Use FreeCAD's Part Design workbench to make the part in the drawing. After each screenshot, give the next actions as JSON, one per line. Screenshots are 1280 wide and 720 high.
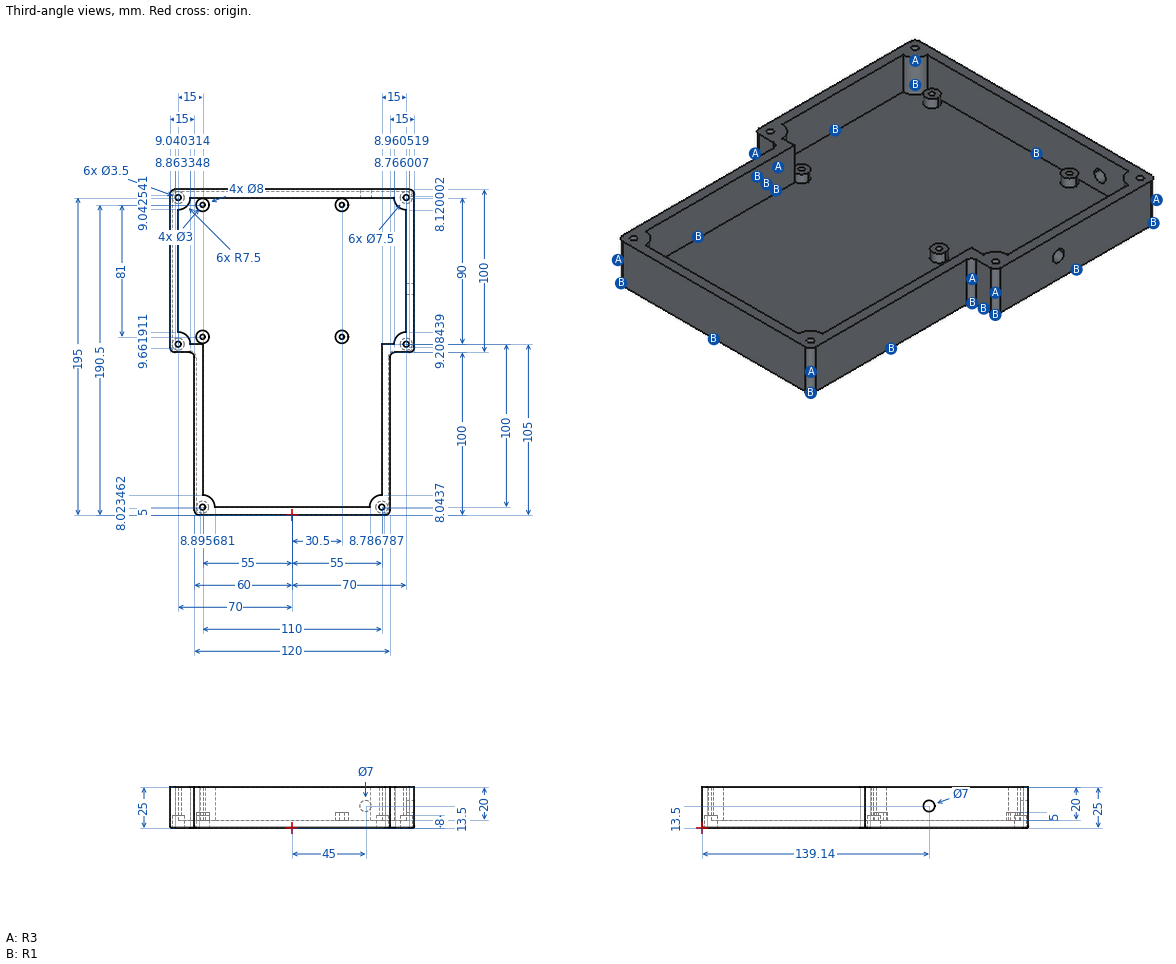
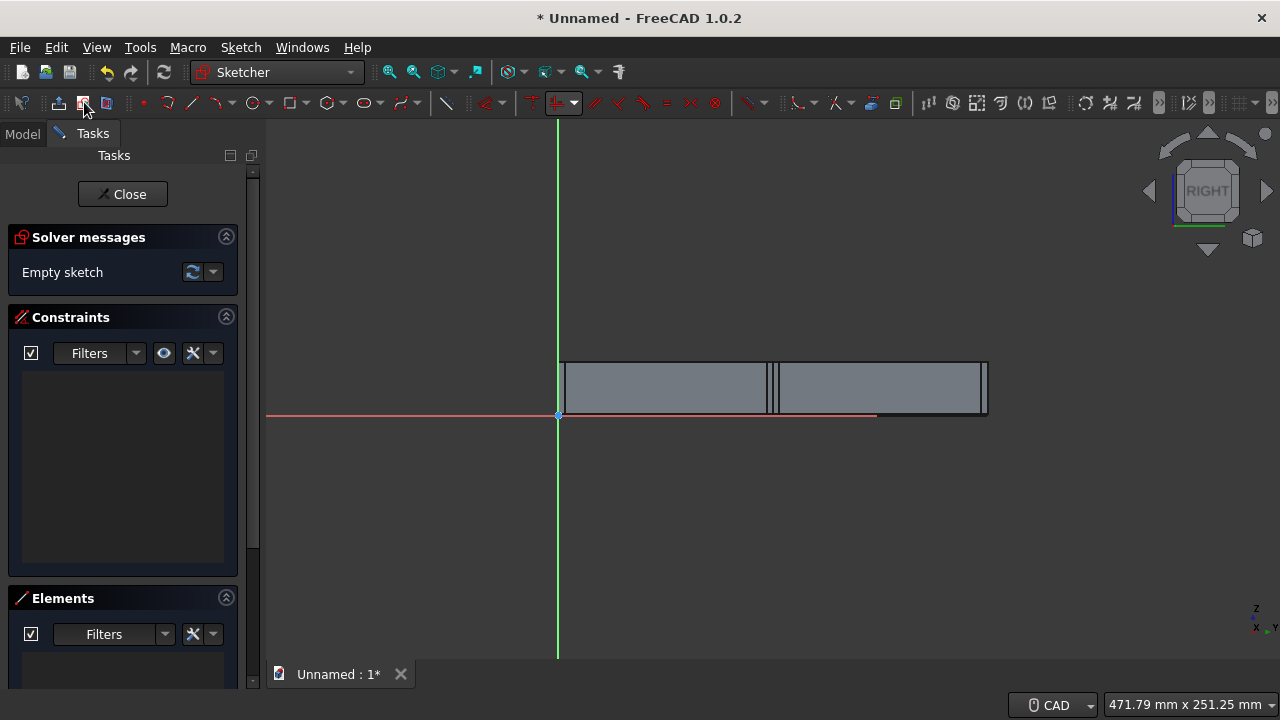
{"action": "scroll", "coordinate": [865, 387], "scroll_direction": "up", "scroll_amount": 15}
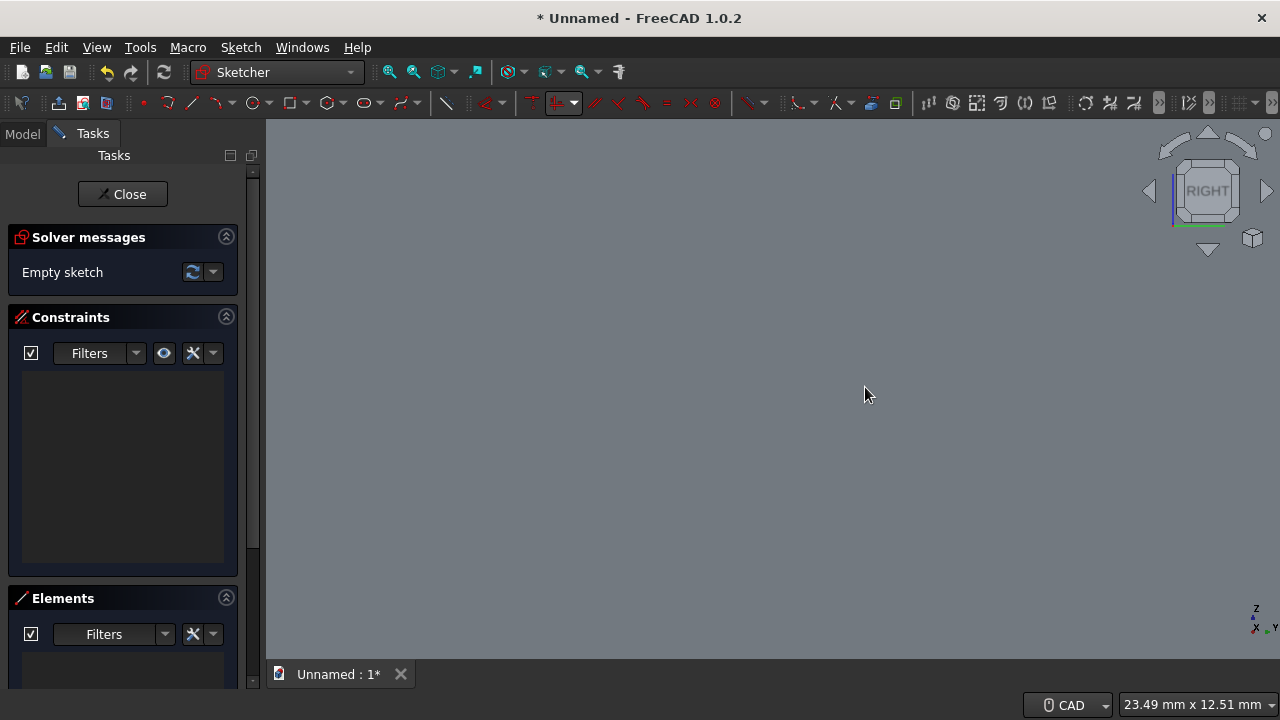
{"action": "left_click", "coordinate": [254, 104]}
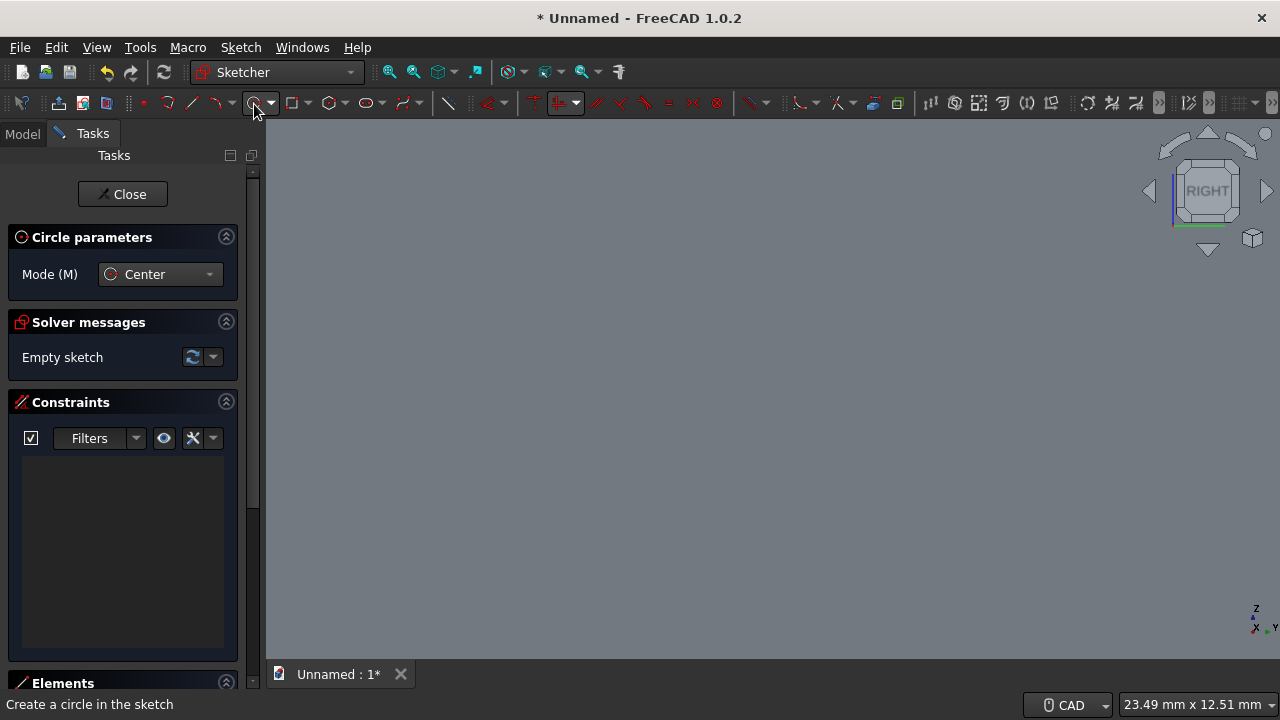
{"action": "left_click", "coordinate": [695, 375]}
{"action": "mouse_move", "coordinate": [802, 268]}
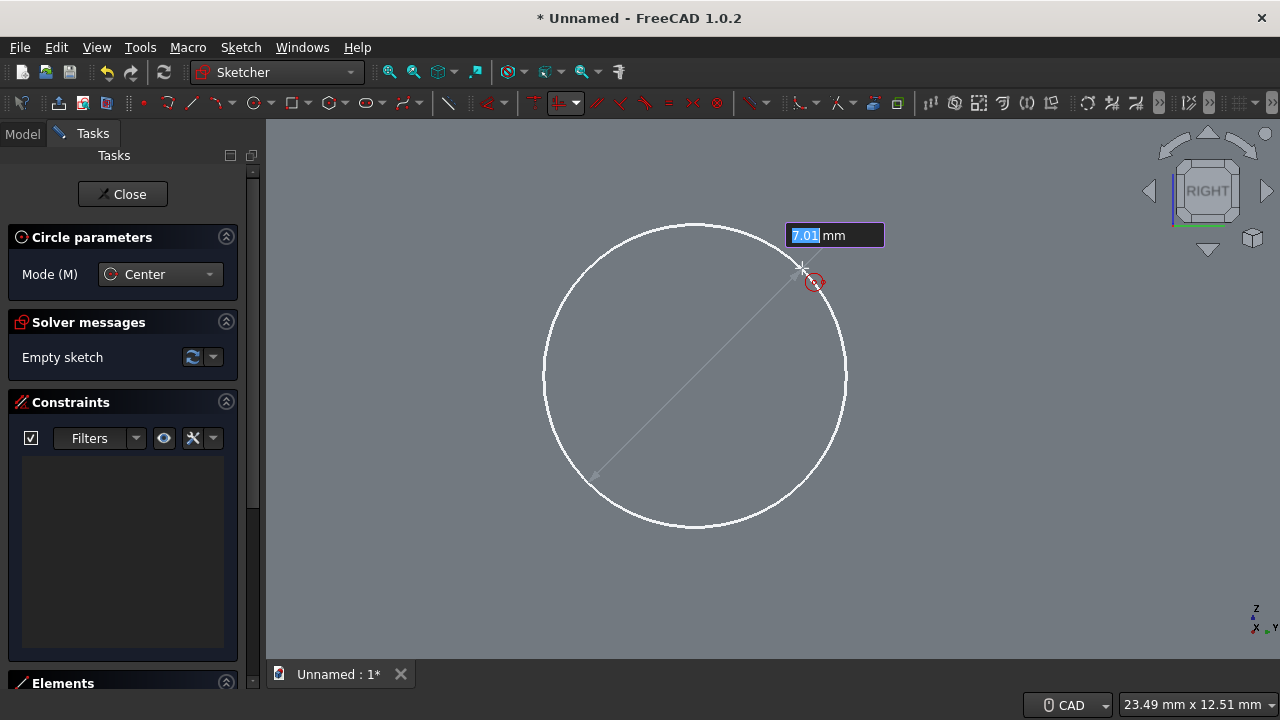
{"action": "type", "text": "7"}
{"action": "key", "text": "Return"}
{"action": "key", "text": "Escape"}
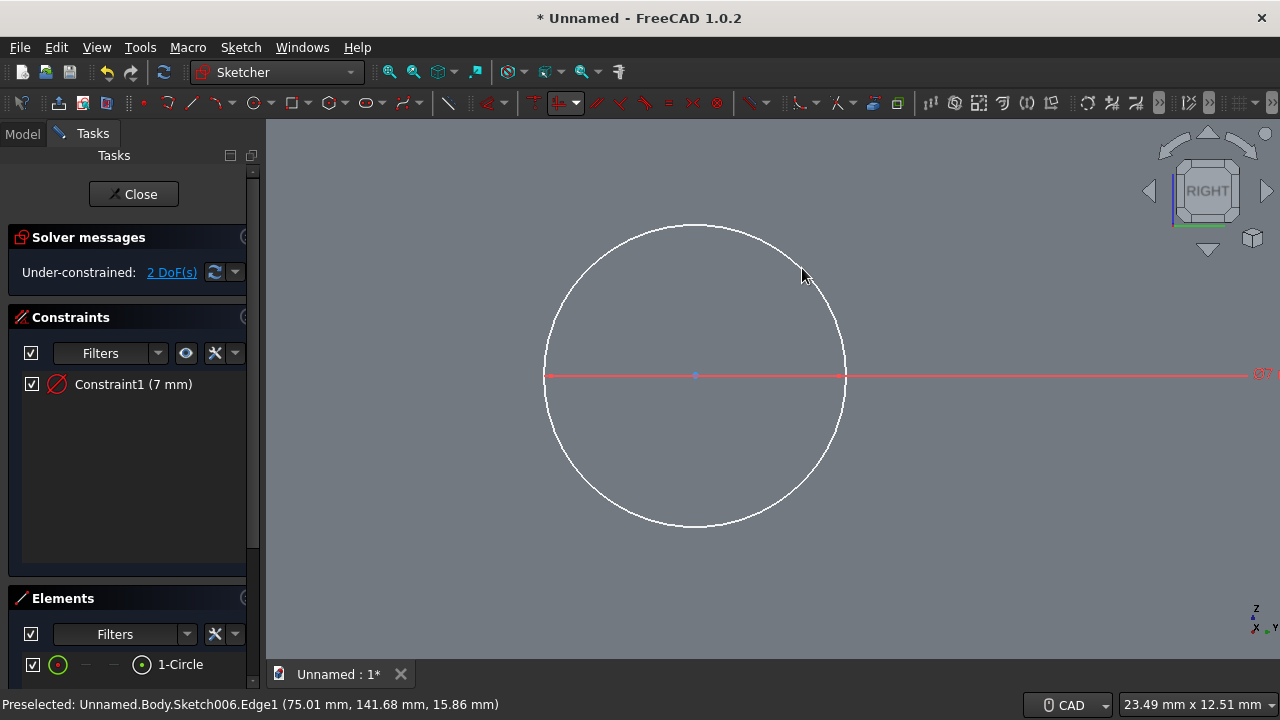
{"action": "left_click", "coordinate": [488, 104]}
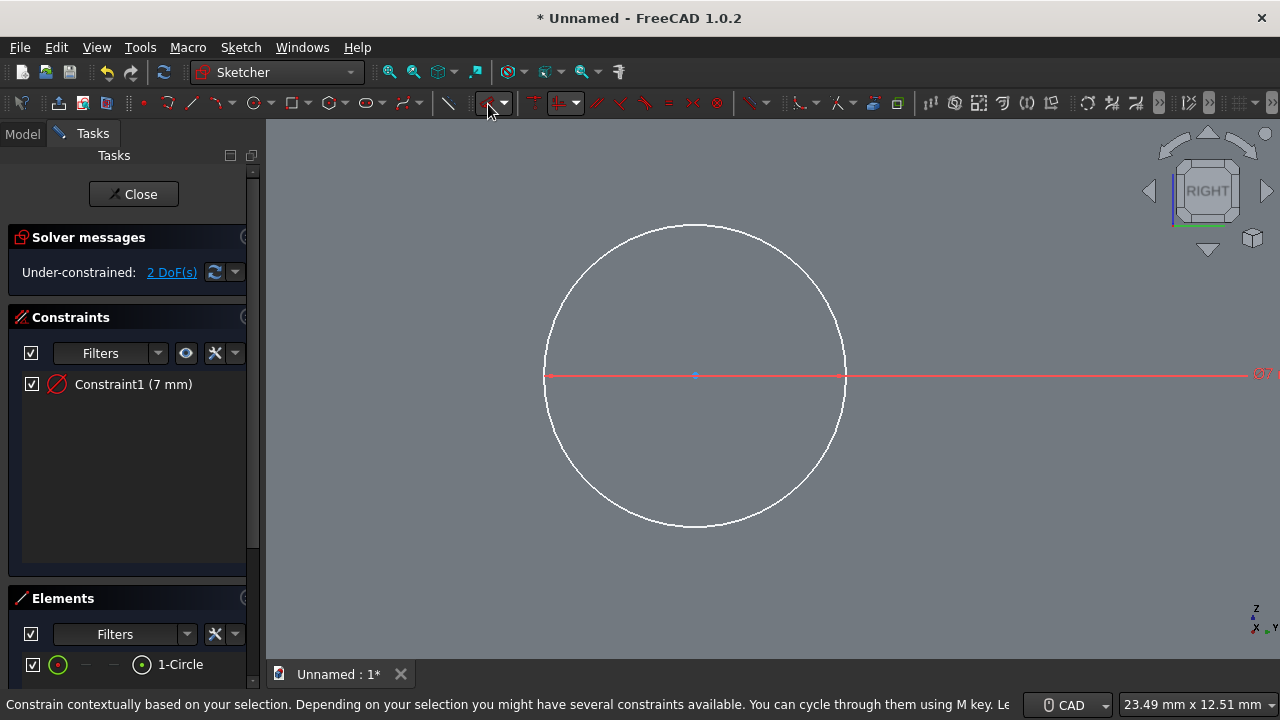
{"action": "left_click", "coordinate": [695, 376]}
{"action": "left_click", "coordinate": [729, 504]}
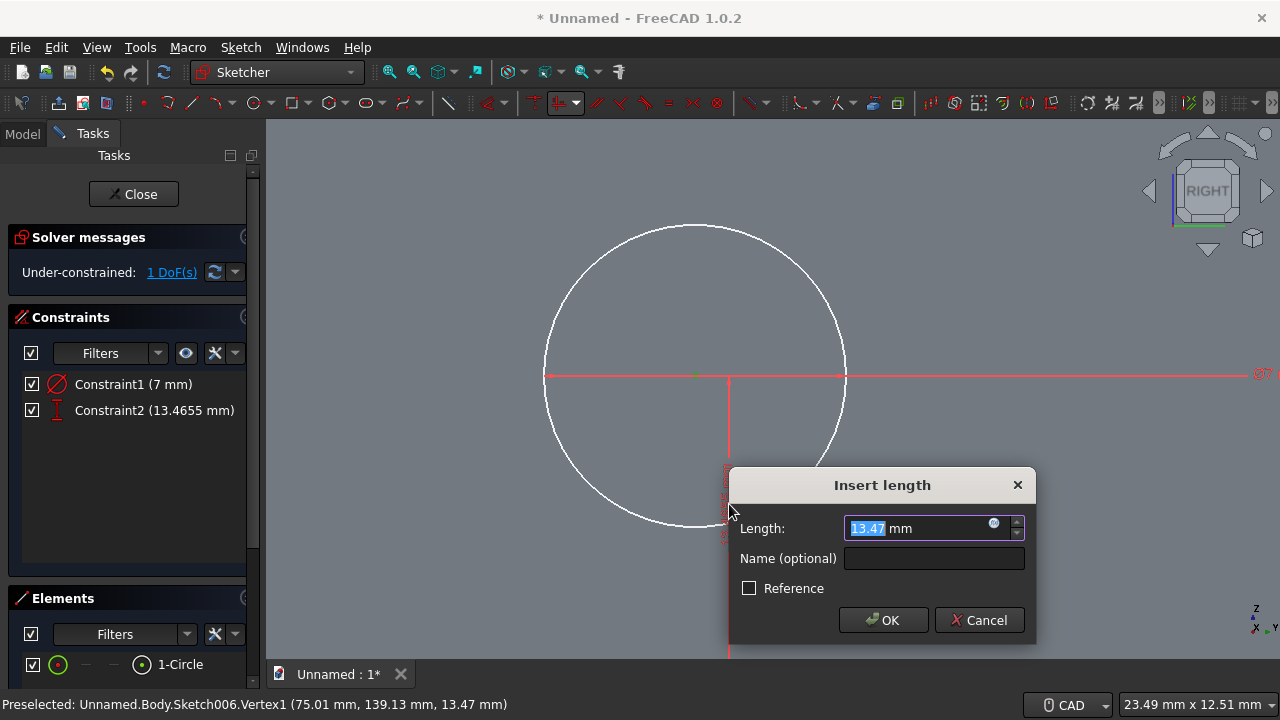
{"action": "type", "text": "13.5"}
{"action": "key", "text": "Return"}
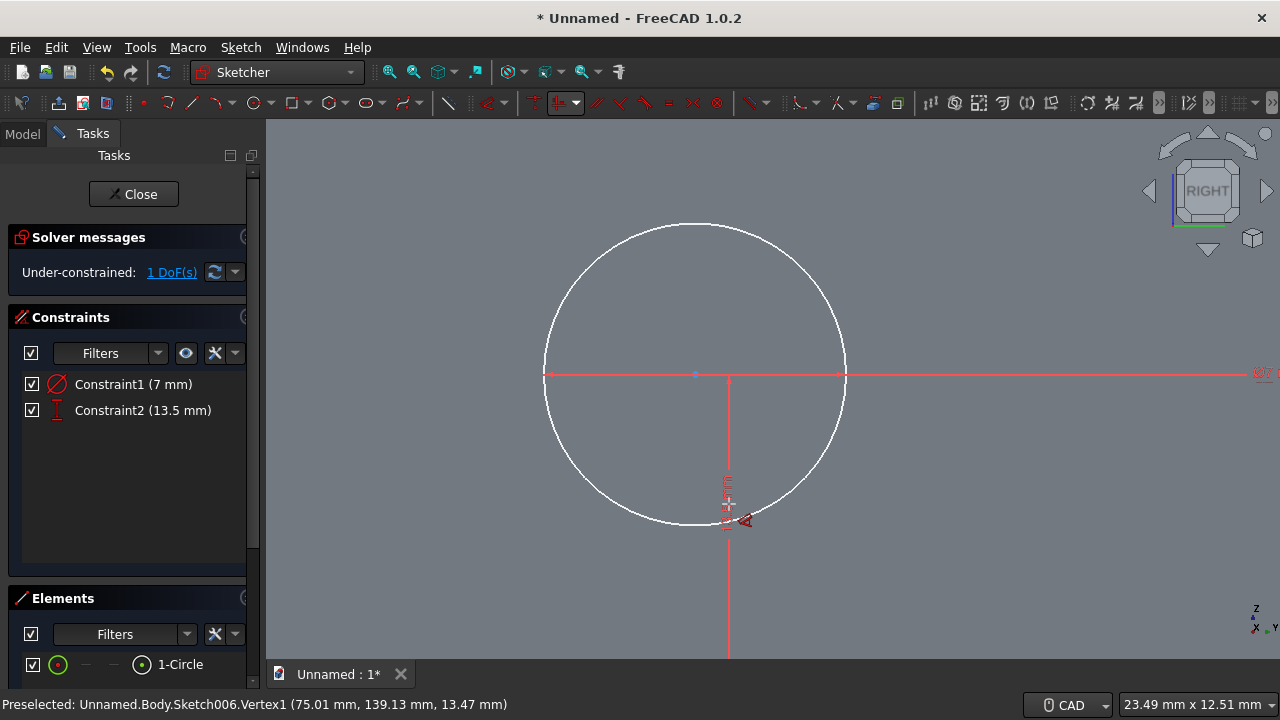
{"action": "left_click", "coordinate": [695, 375]}
{"action": "left_click", "coordinate": [494, 341]}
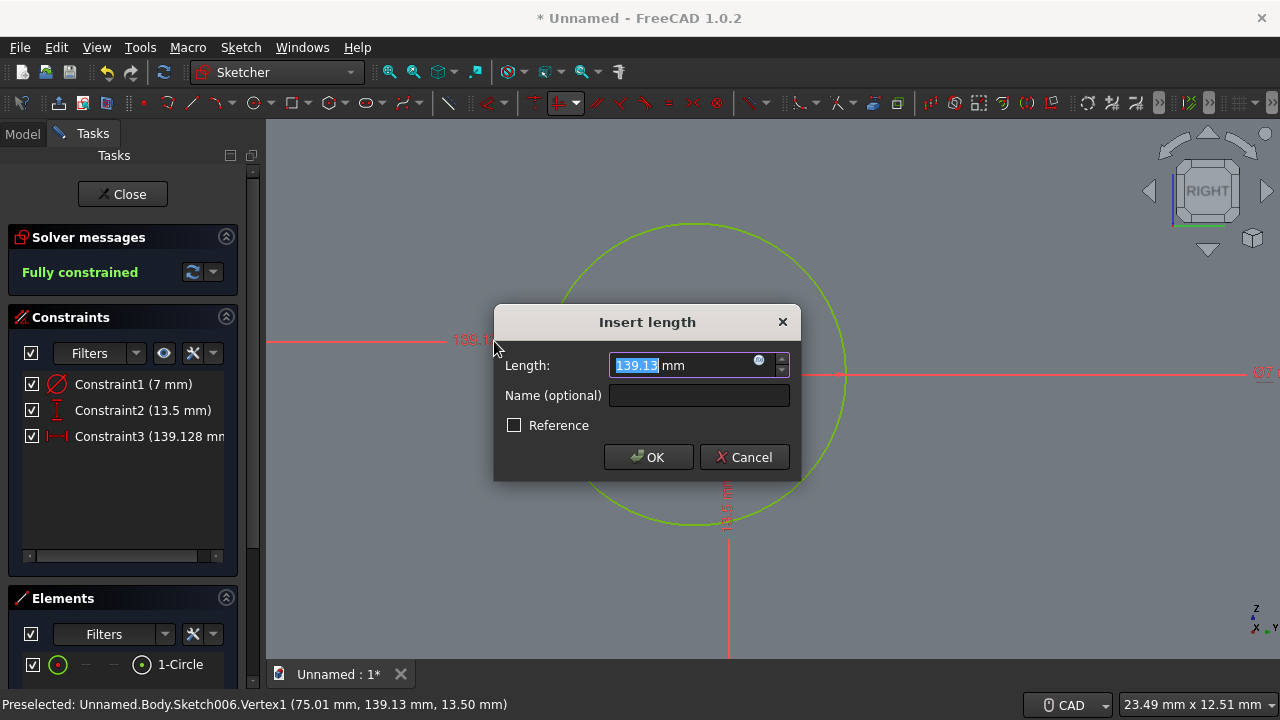
{"action": "type", "text": "139.14"}
{"action": "key", "text": "Return"}
{"action": "key", "text": "Escape"}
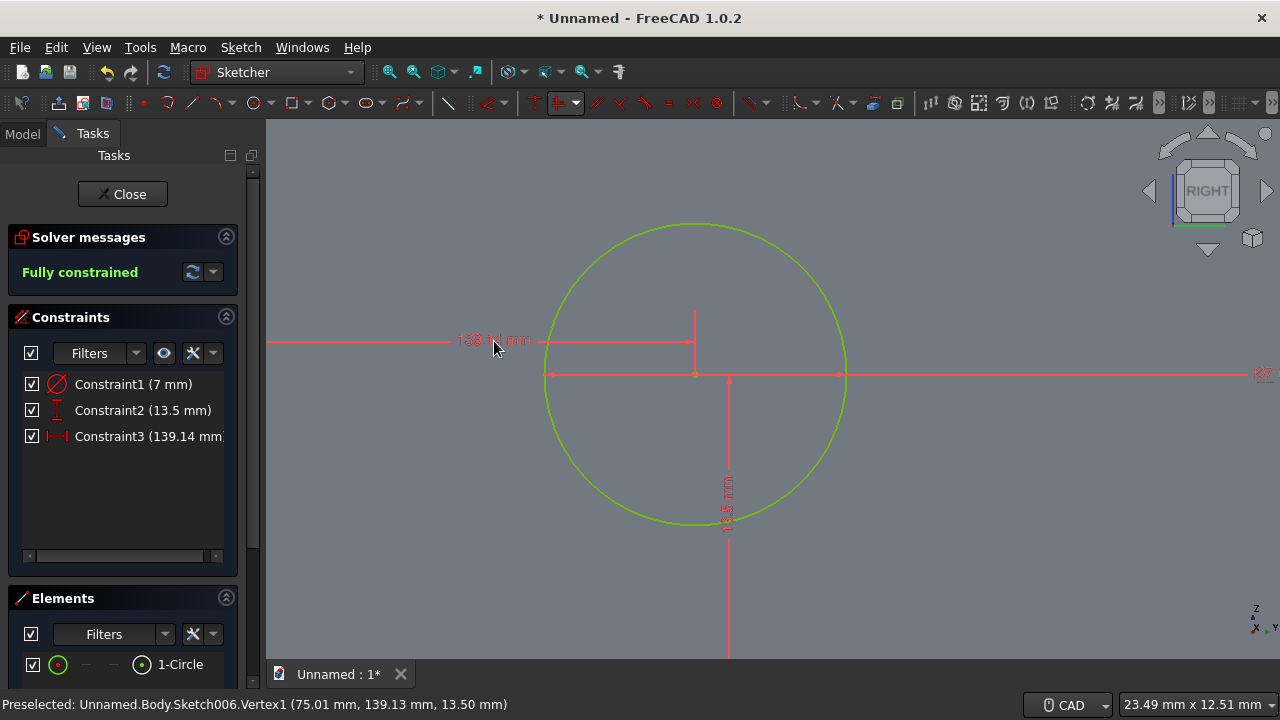
{"action": "left_click", "coordinate": [123, 194]}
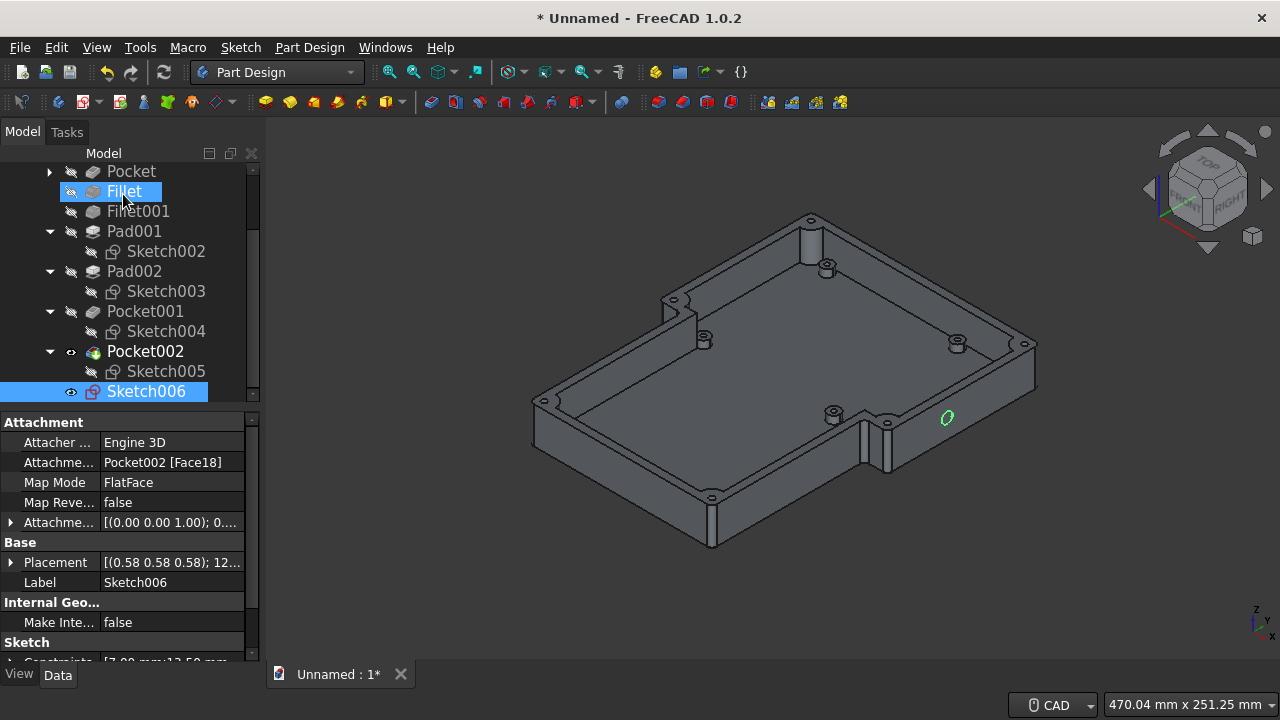
{"action": "left_click", "coordinate": [432, 102]}